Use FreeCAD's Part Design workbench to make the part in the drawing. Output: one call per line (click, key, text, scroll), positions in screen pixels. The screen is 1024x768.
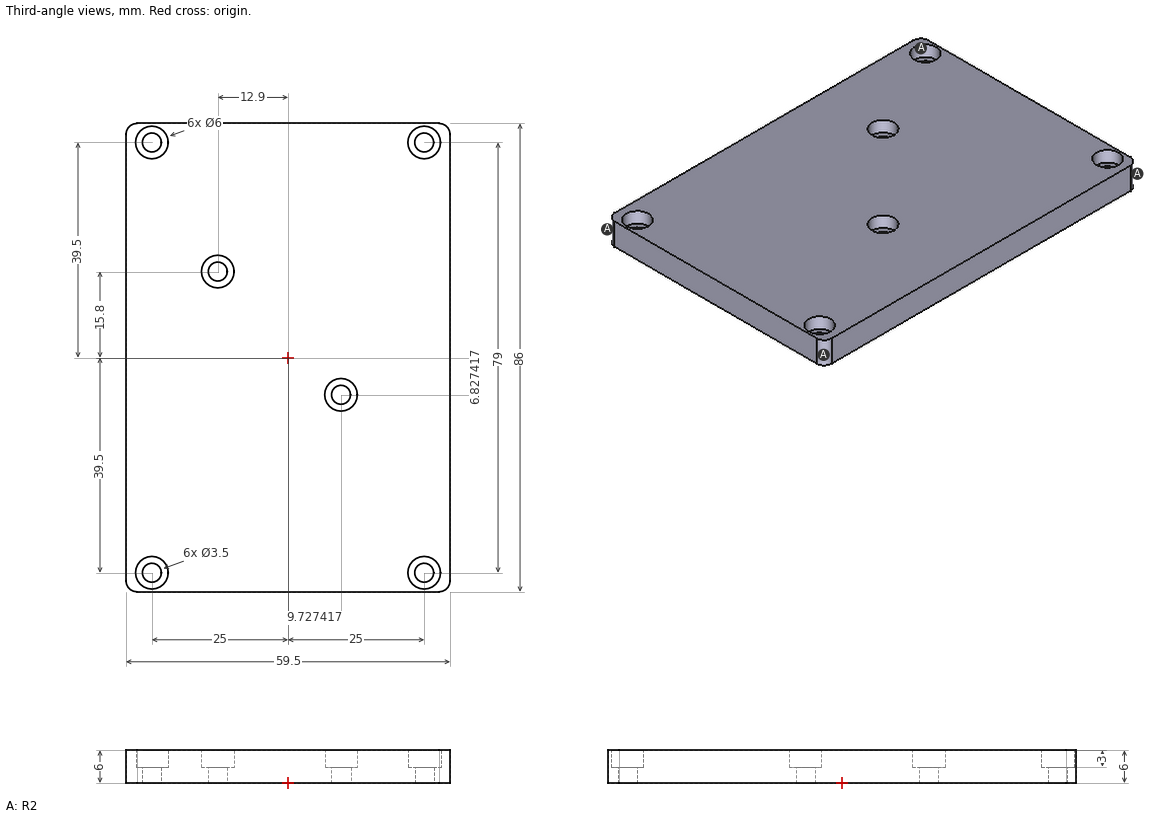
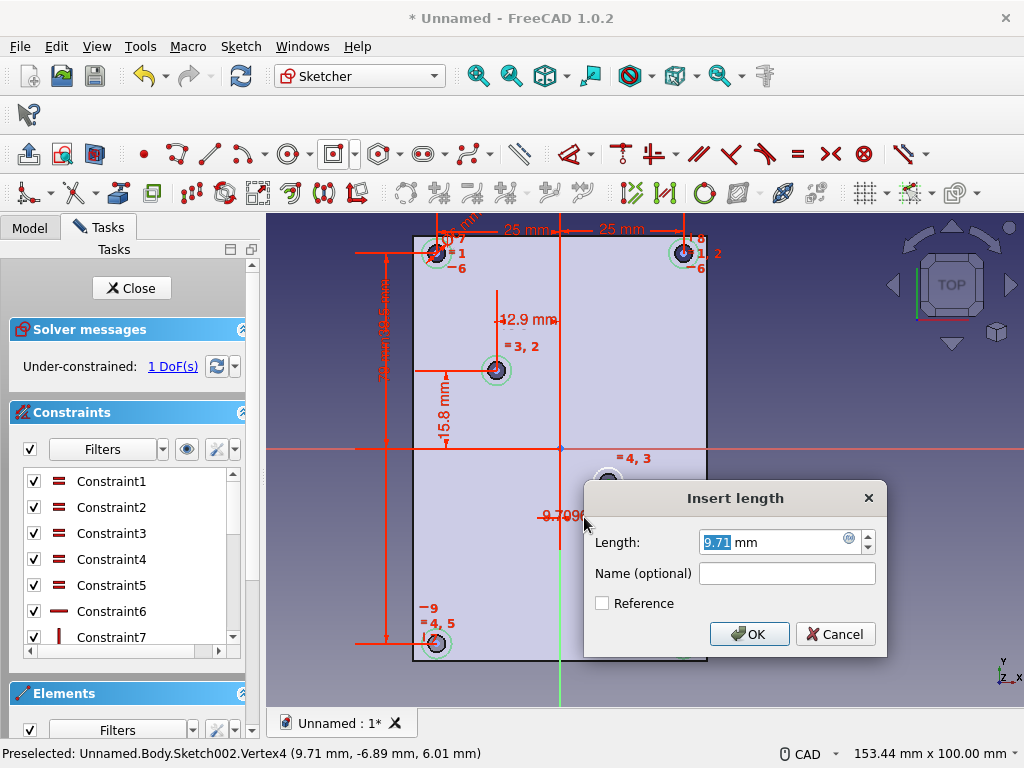
text(9.727417)
key(Return)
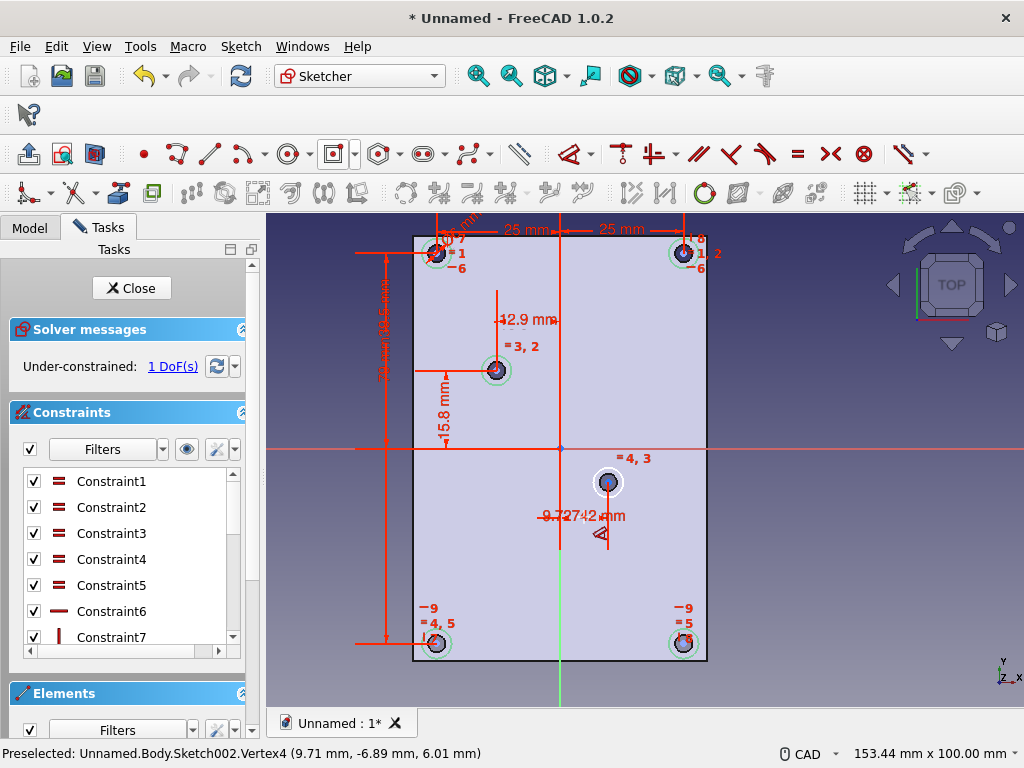
click(608, 483)
click(642, 466)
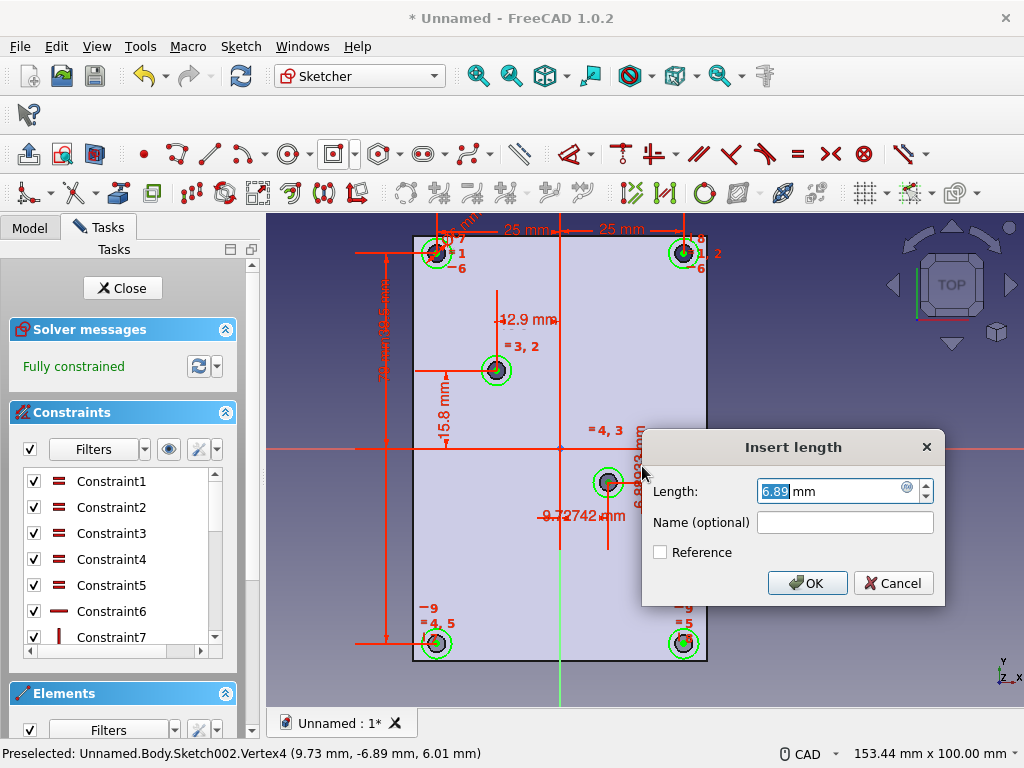
text(6.827417)
key(Return)
key(Escape)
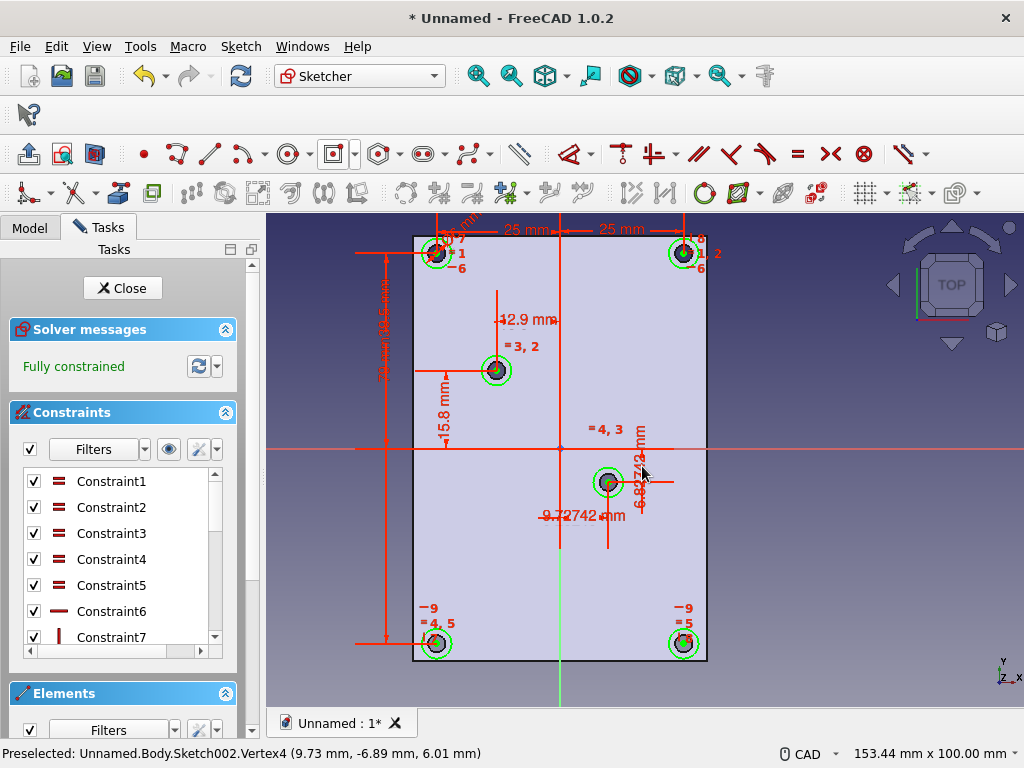
click(123, 288)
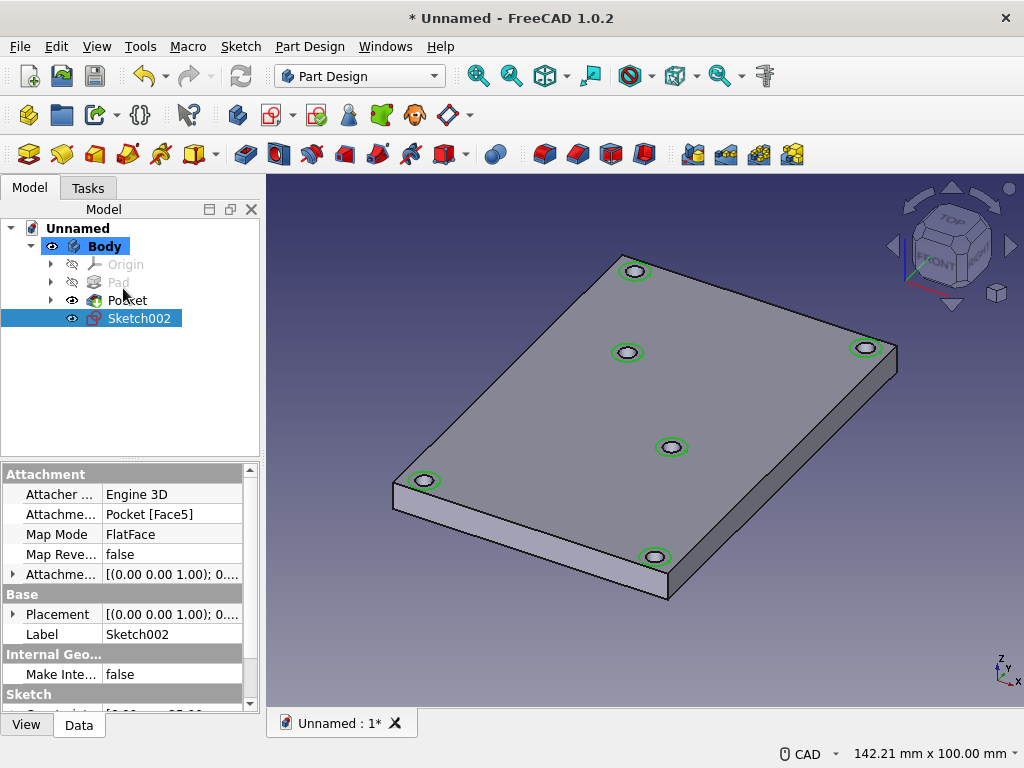
click(246, 154)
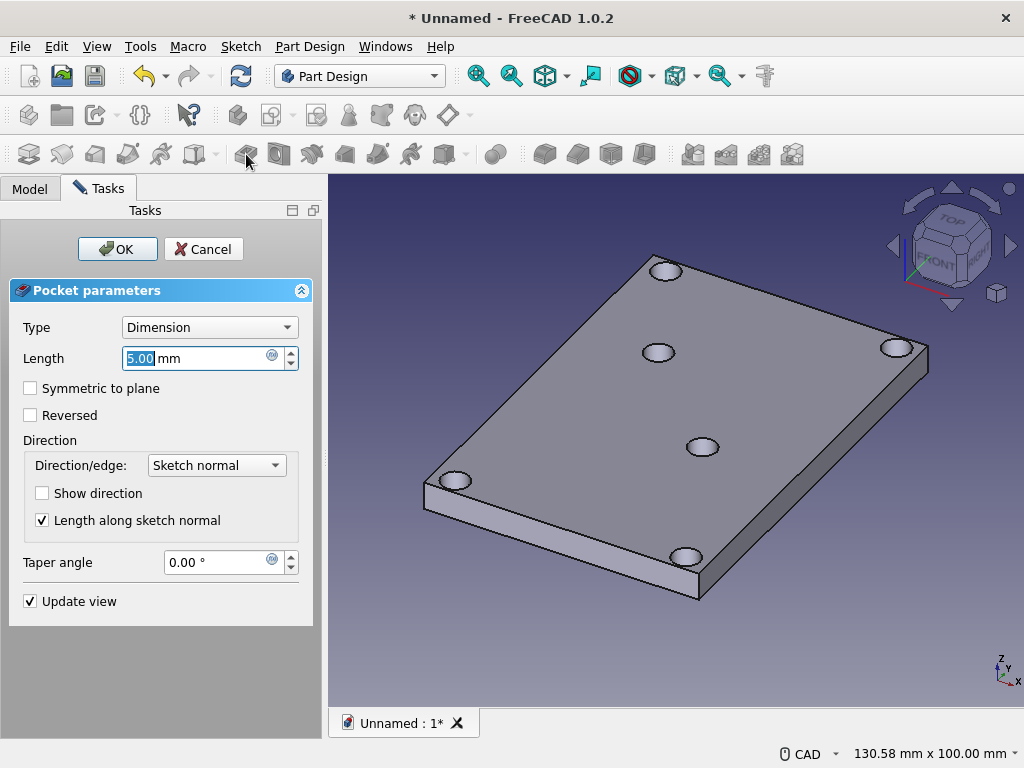
text(3)
key(Tab)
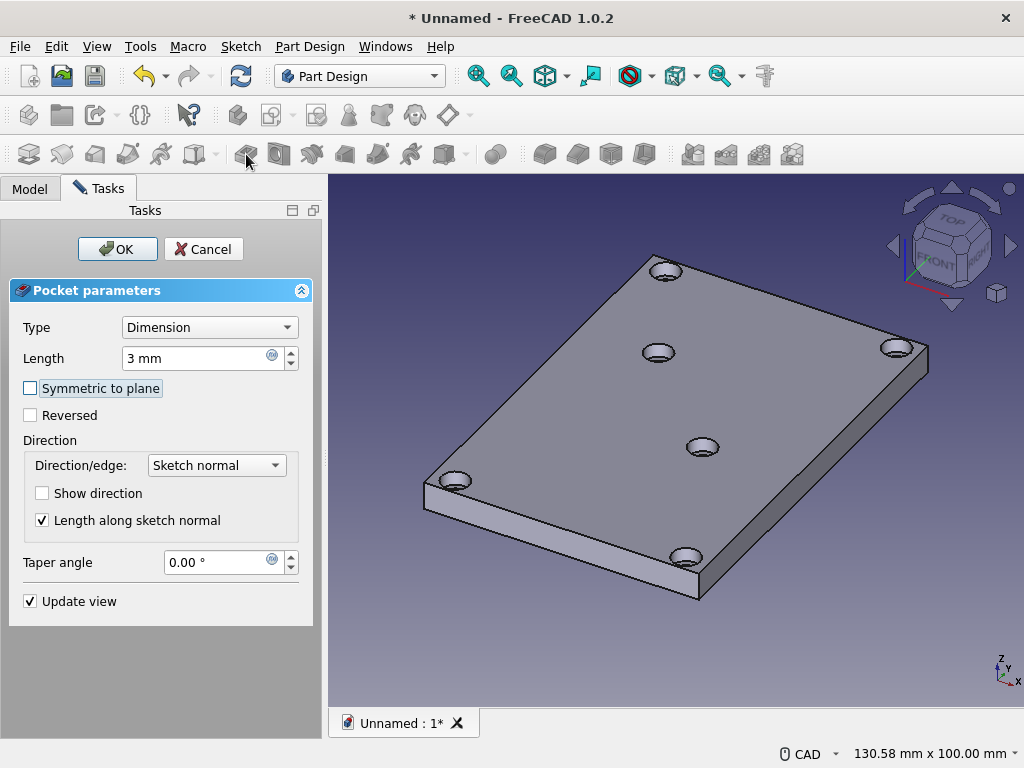
click(118, 249)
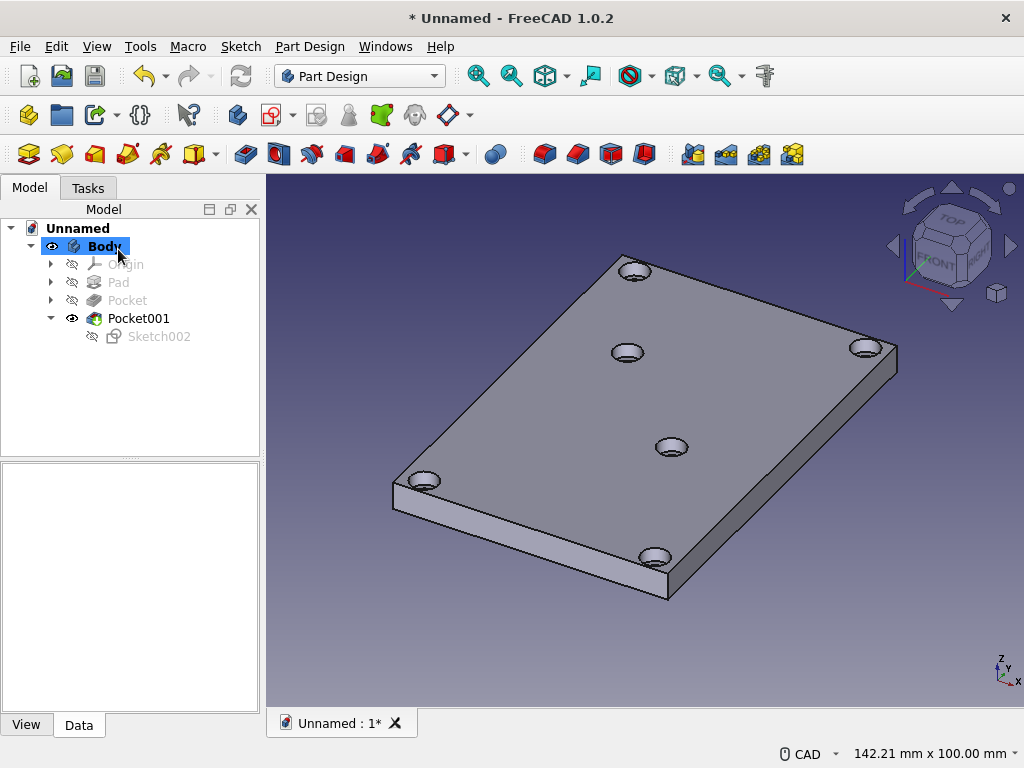
click(668, 586)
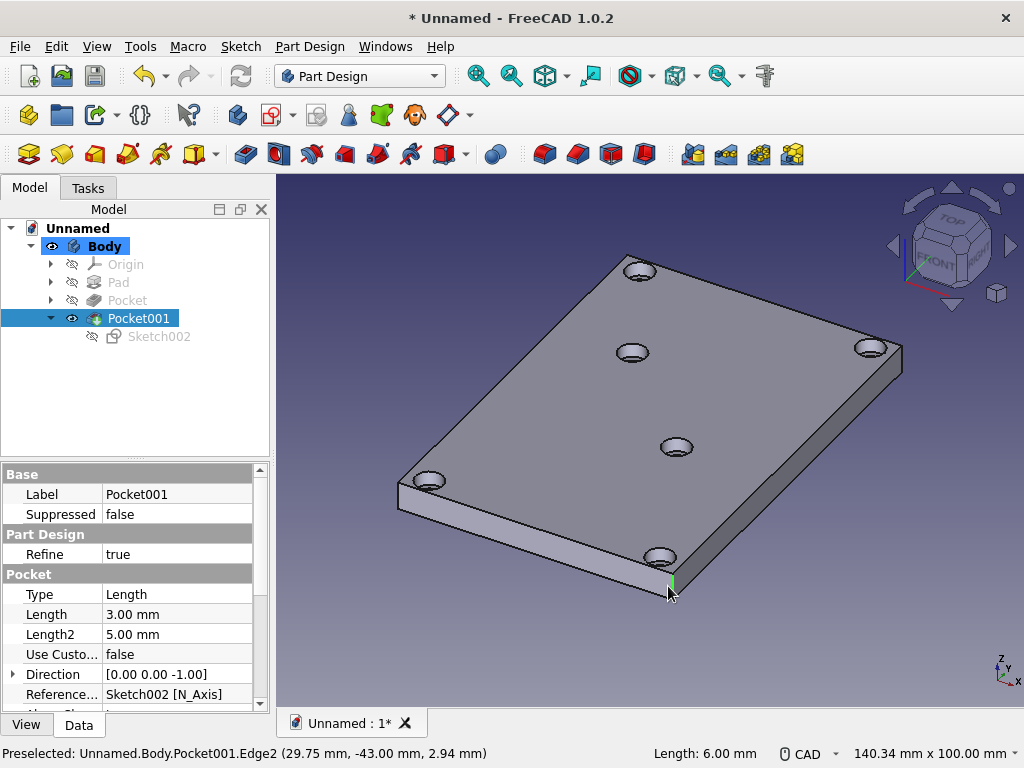
key(0)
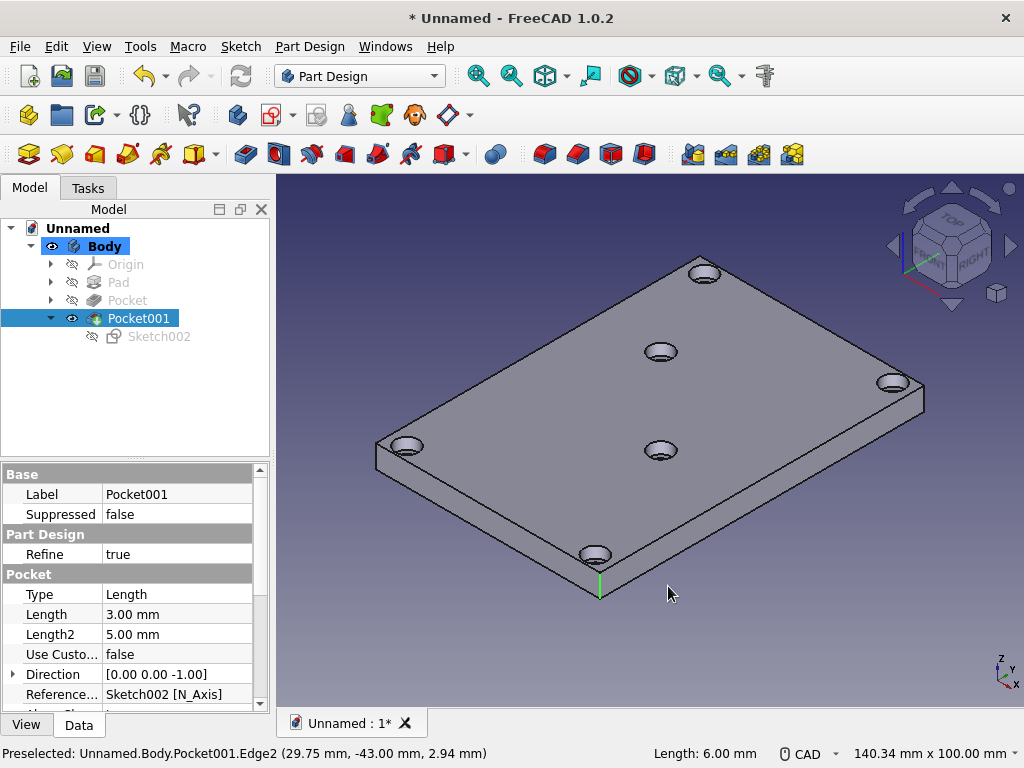
key(2)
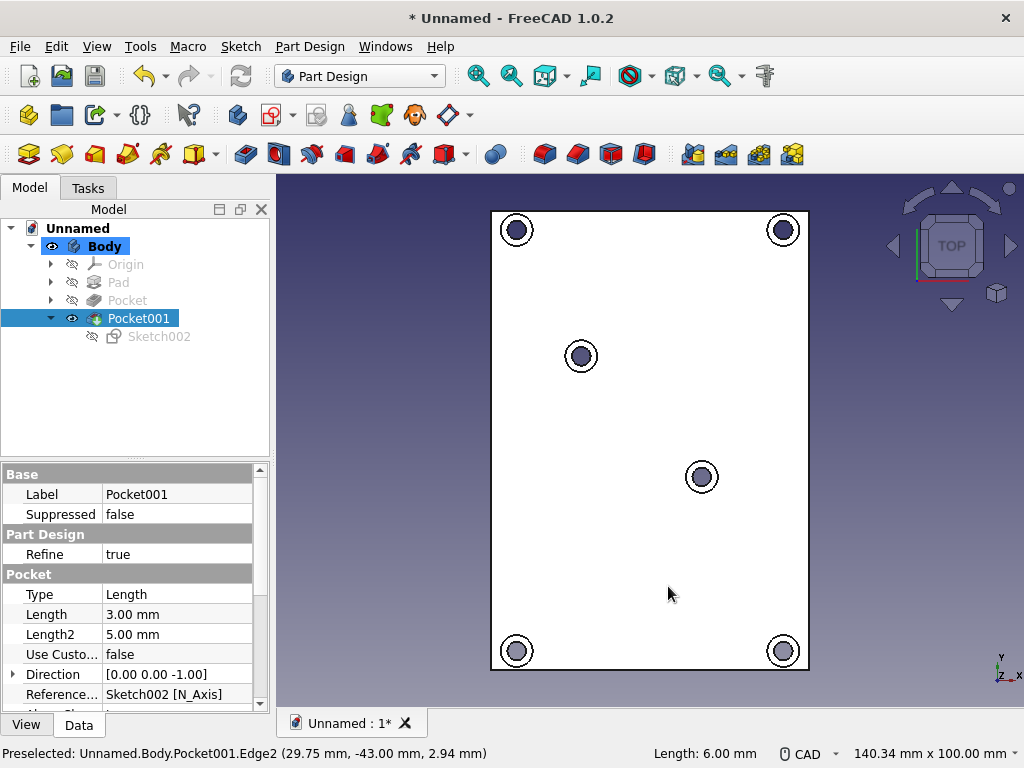
key(1)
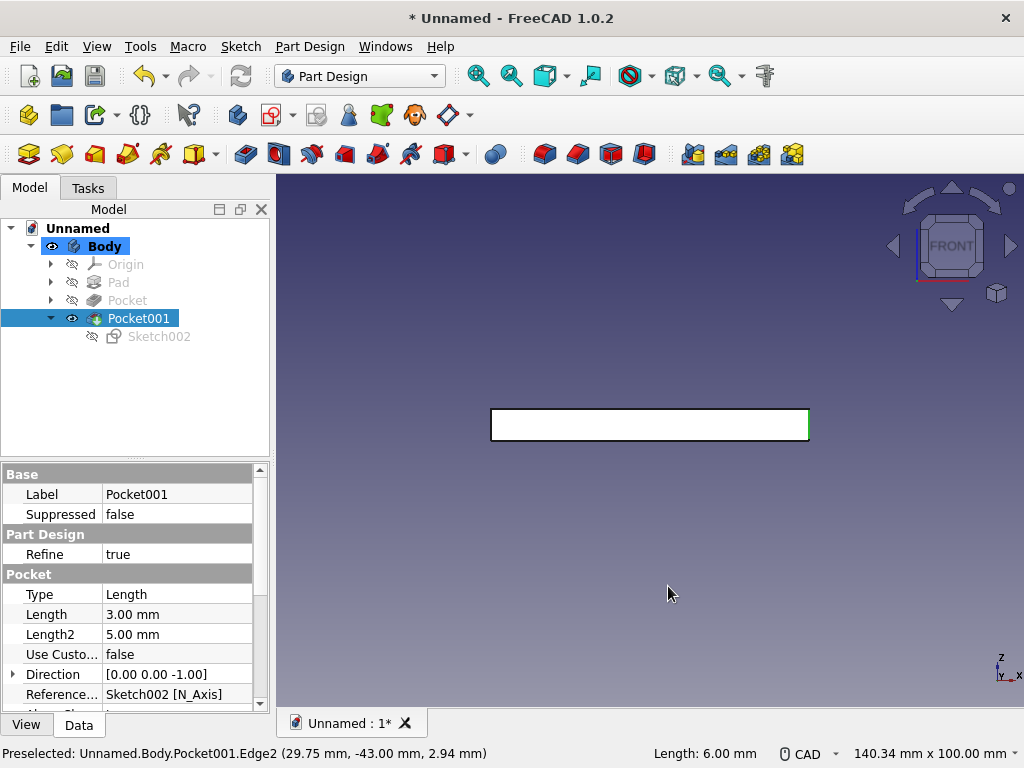
key(v)
key(f)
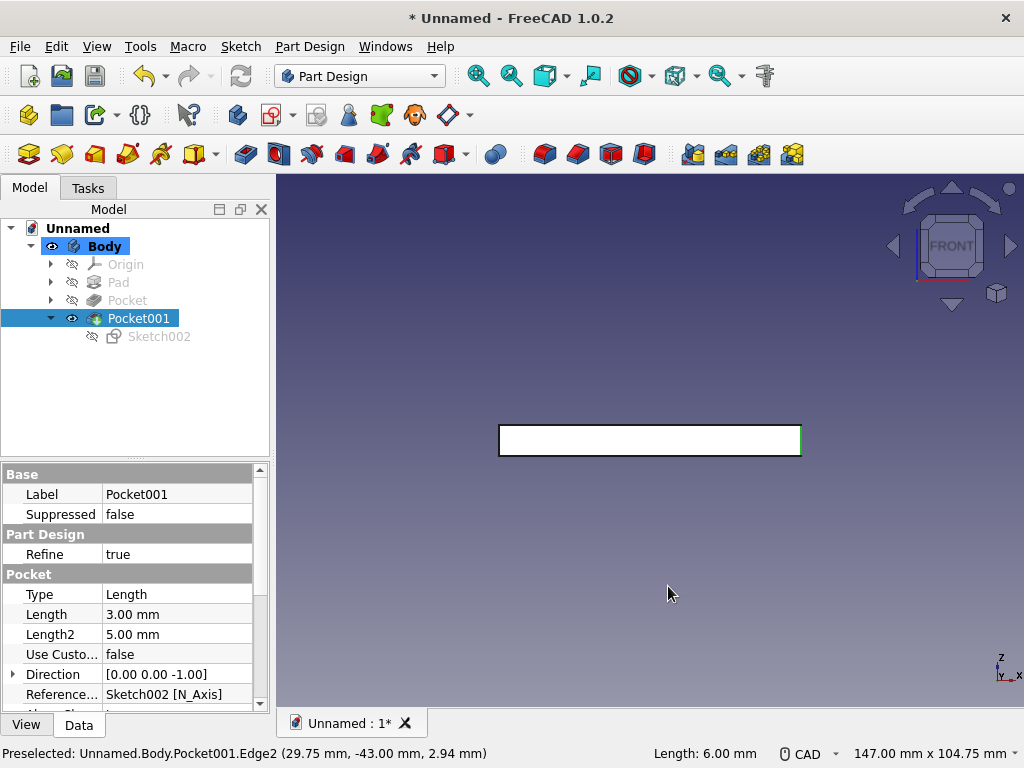
click(499, 440, ctrl)